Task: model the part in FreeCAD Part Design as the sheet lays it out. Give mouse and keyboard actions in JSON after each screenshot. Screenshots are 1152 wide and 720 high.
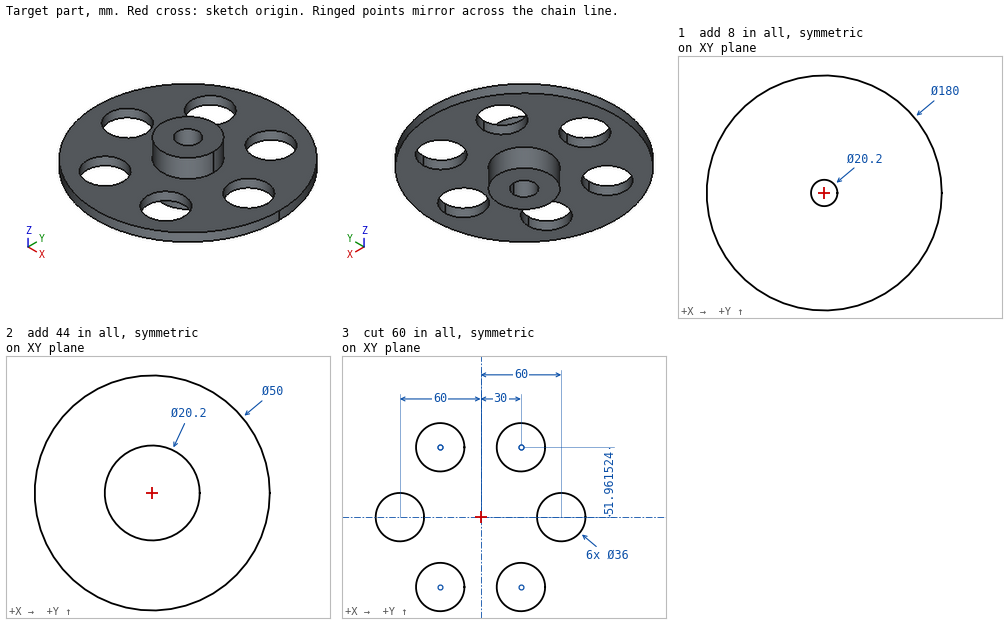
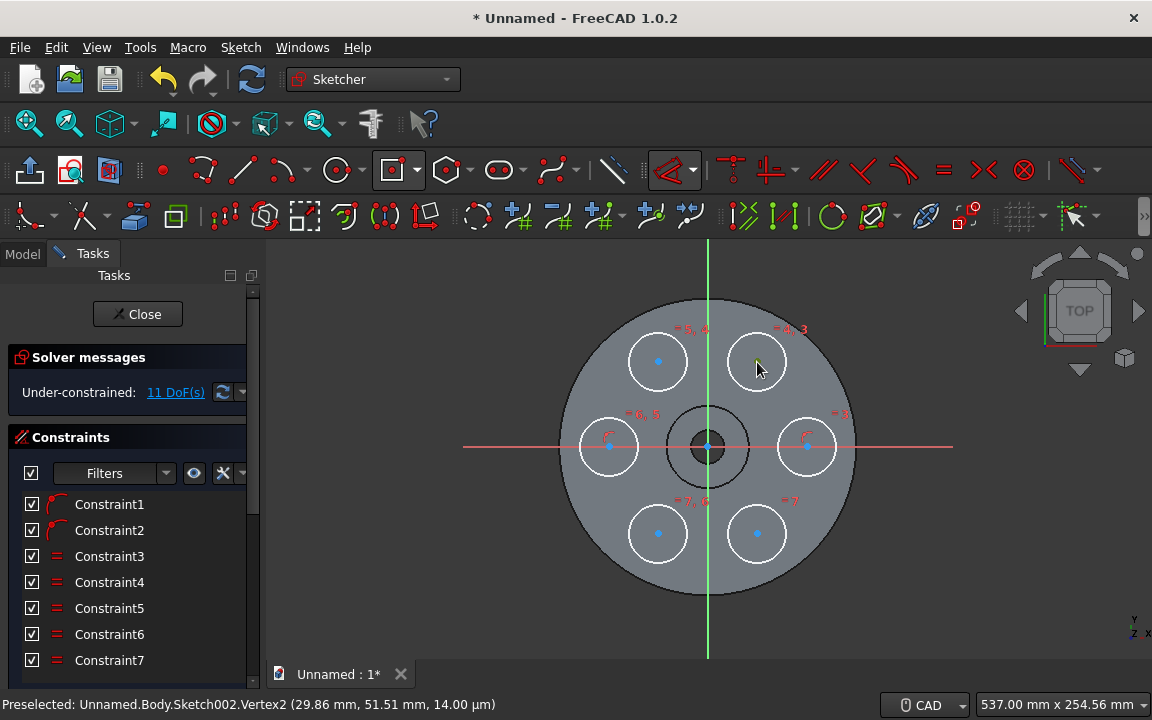
{"action": "left_click", "coordinate": [658, 362]}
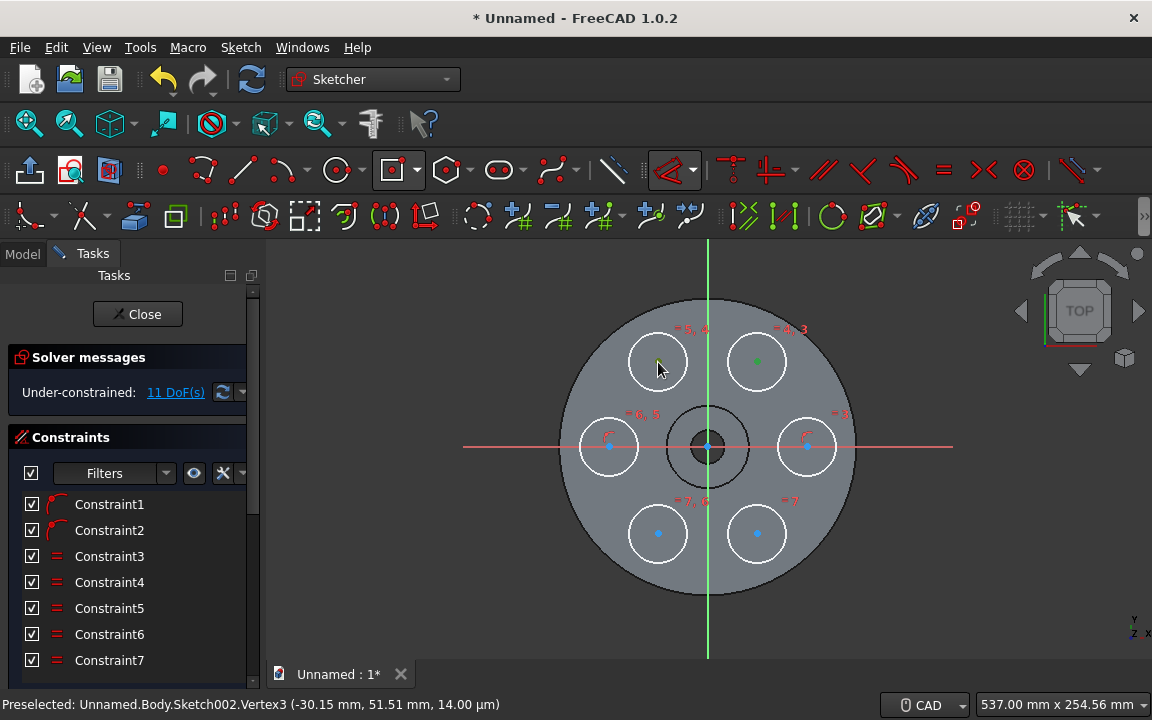
{"action": "left_click", "coordinate": [708, 605]}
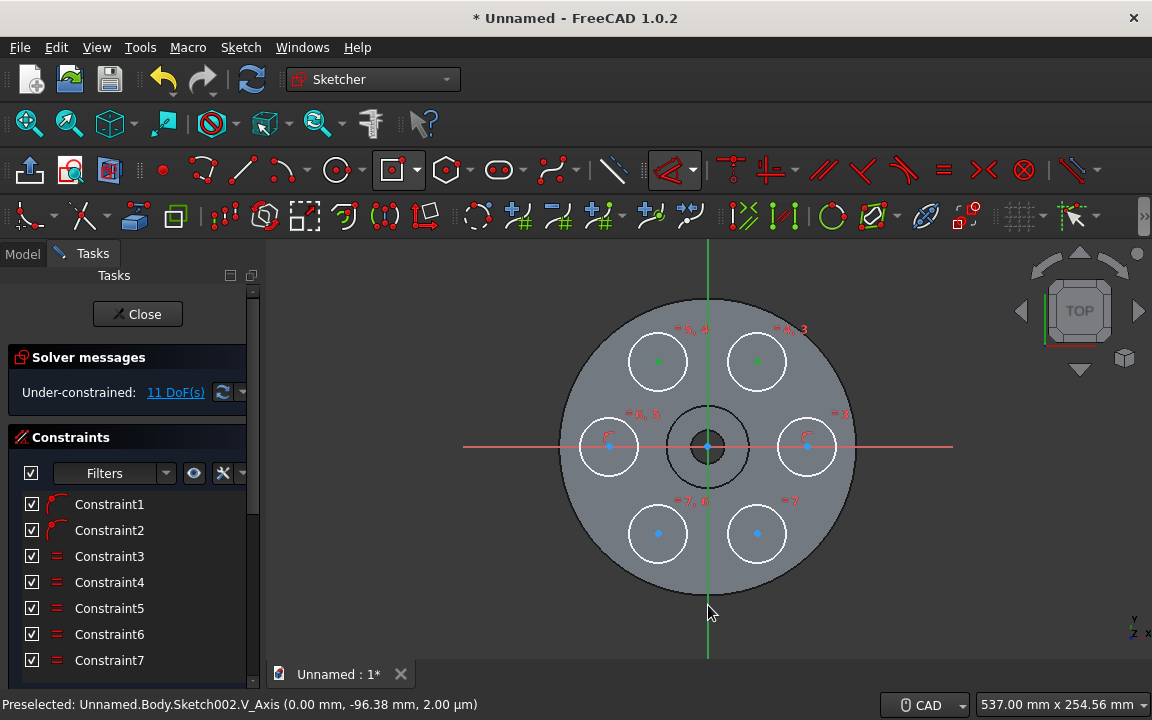
{"action": "key", "text": "s"}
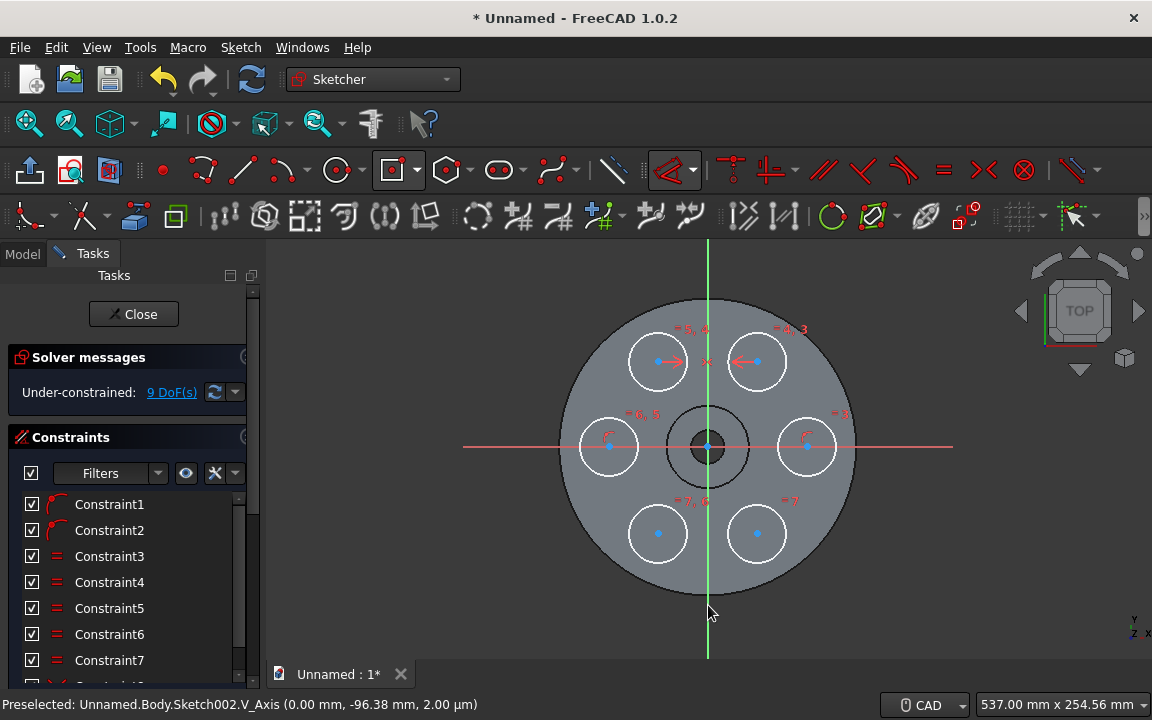
{"action": "left_click", "coordinate": [658, 362]}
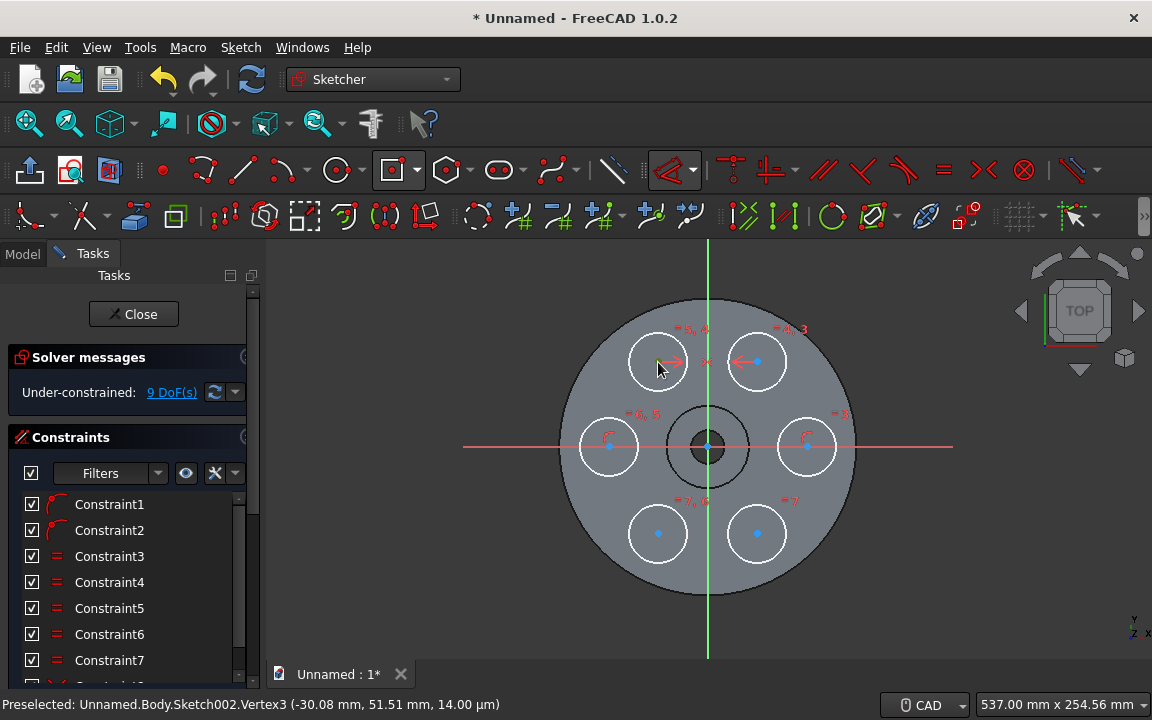
{"action": "left_click", "coordinate": [658, 534]}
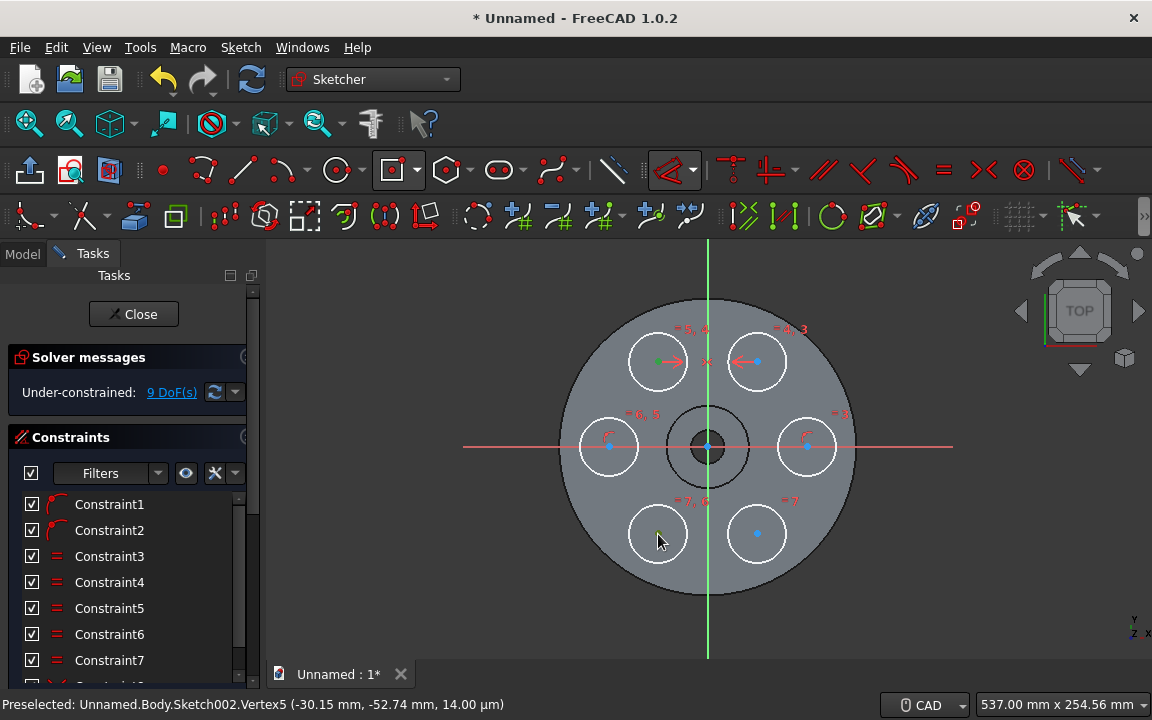
{"action": "left_click", "coordinate": [492, 447]}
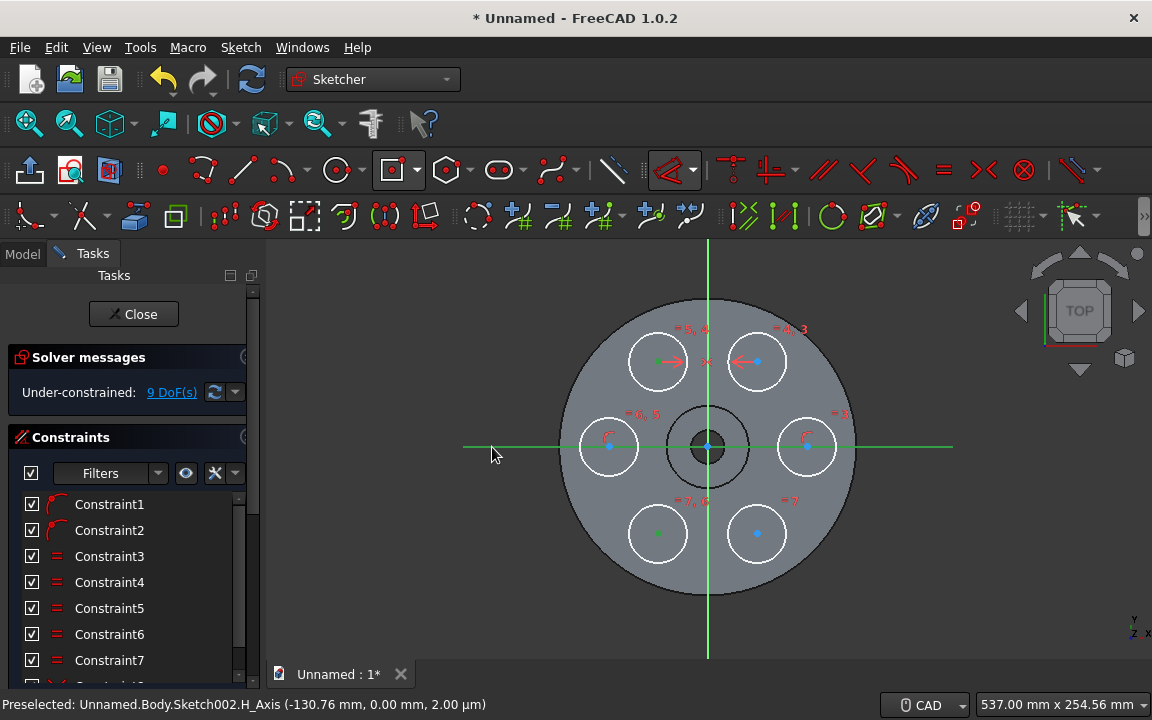
{"action": "key", "text": "s"}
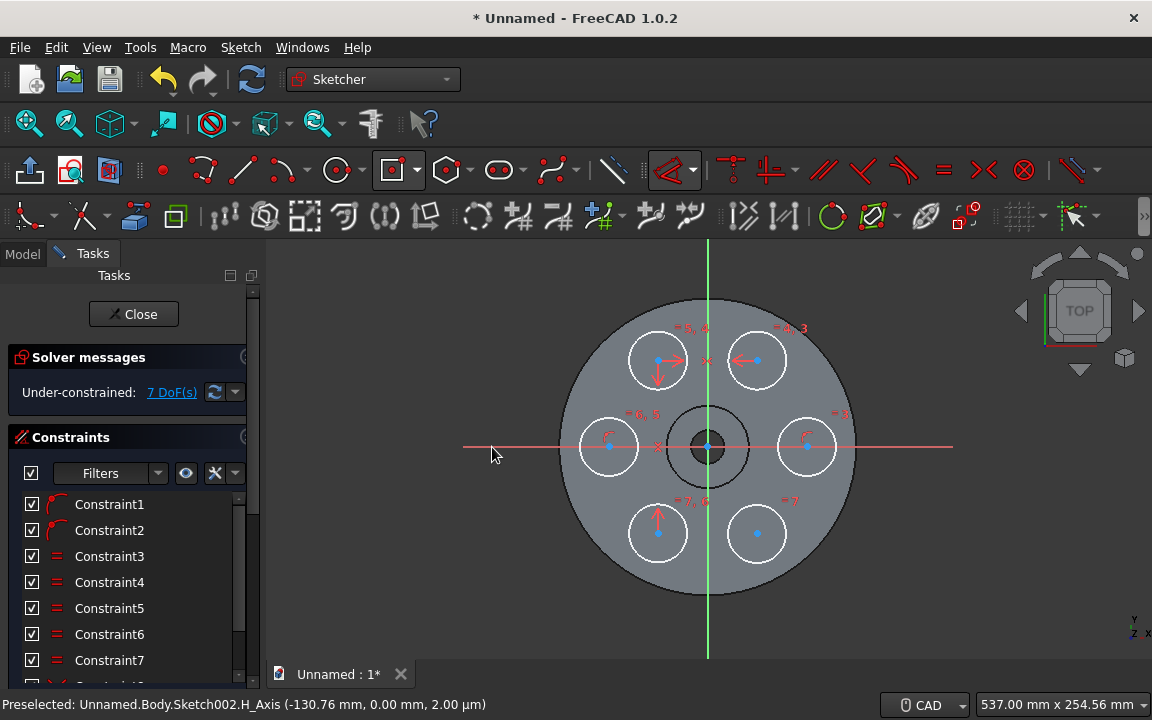
{"action": "left_click", "coordinate": [757, 361]}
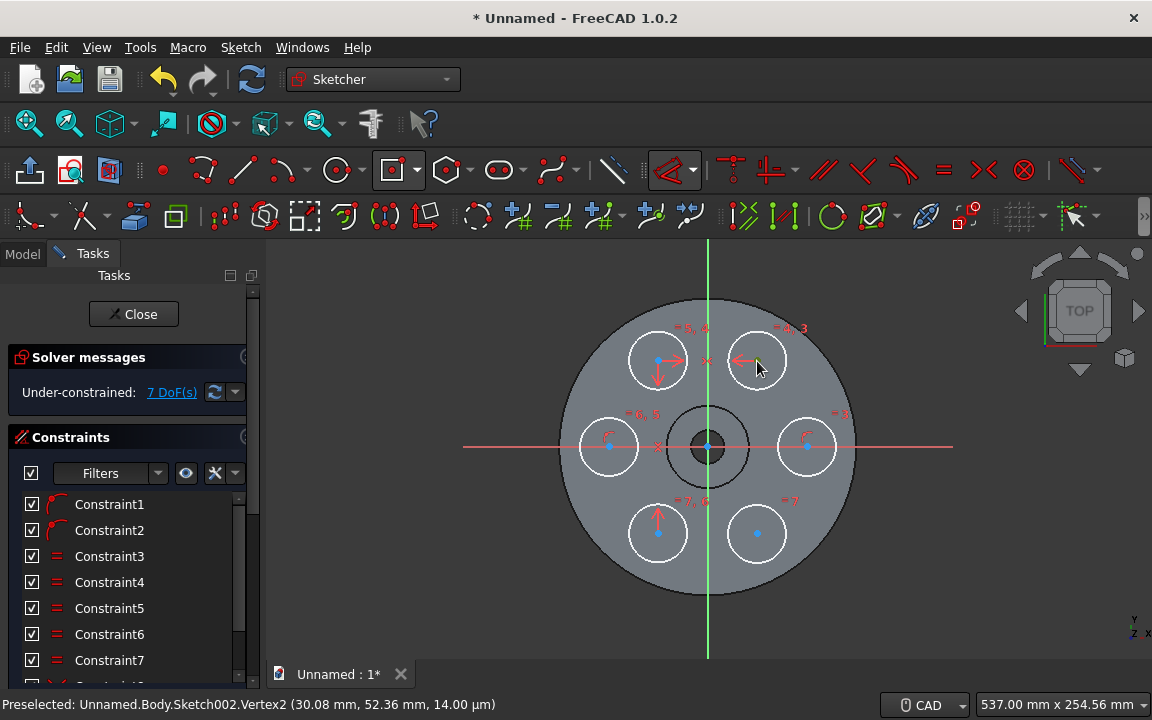
{"action": "left_click", "coordinate": [757, 534]}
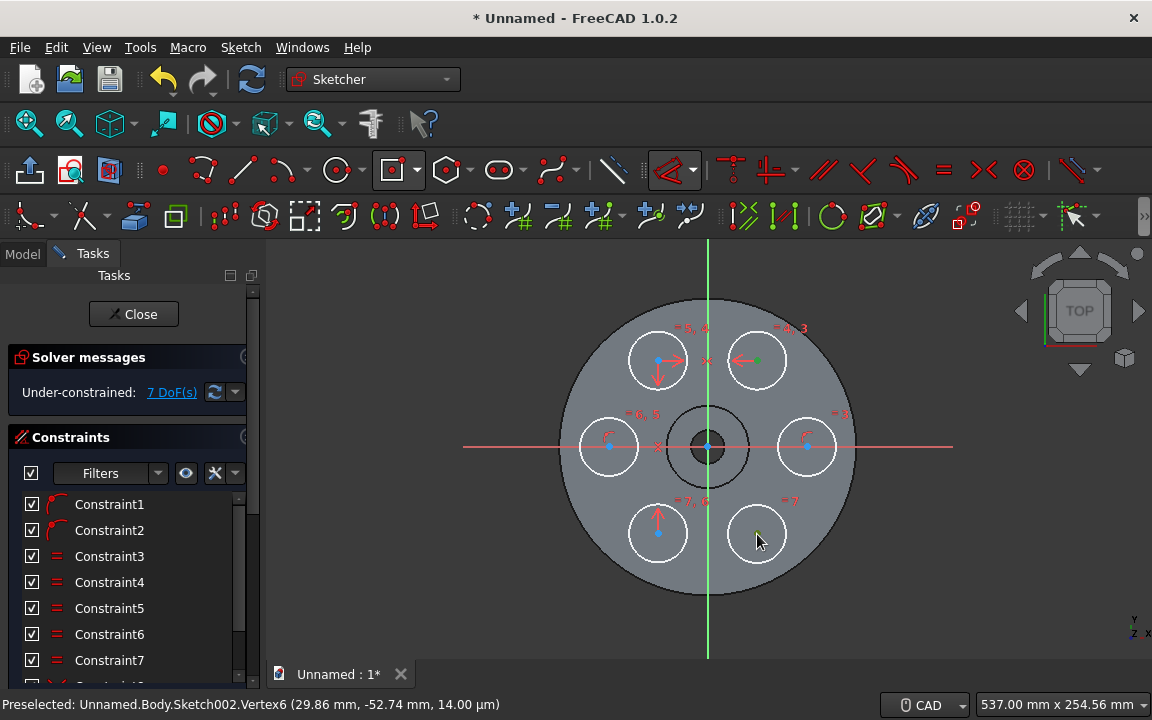
{"action": "left_click", "coordinate": [492, 447]}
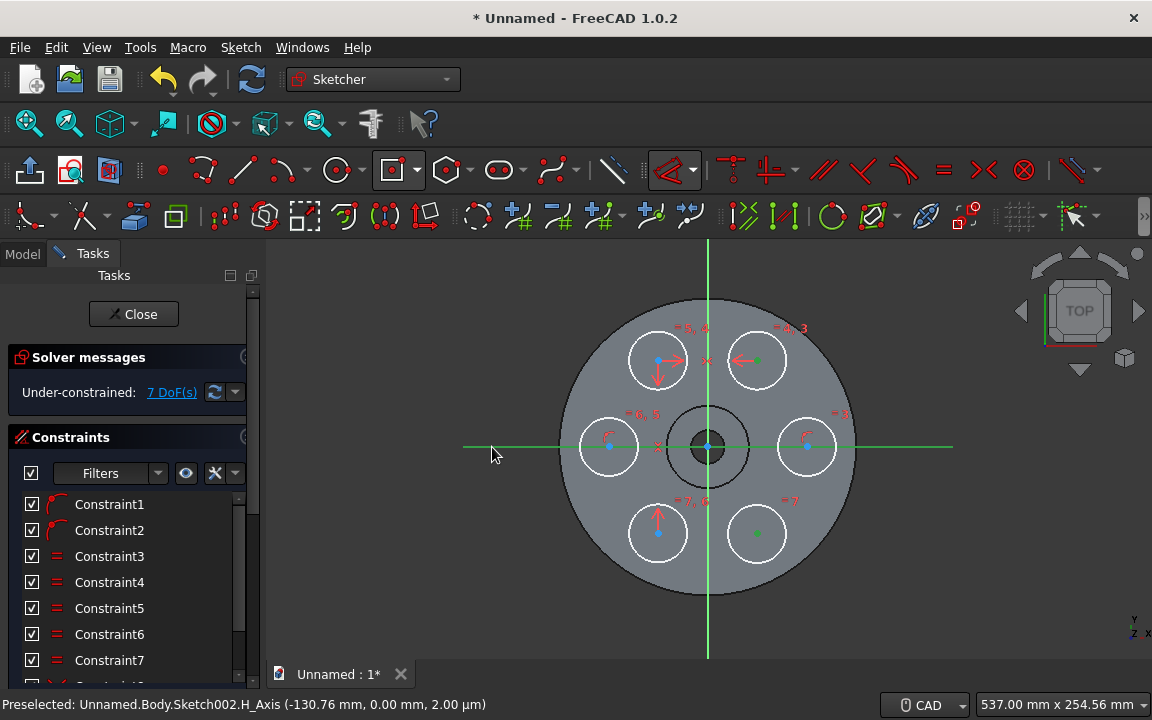
{"action": "left_click", "coordinate": [984, 170]}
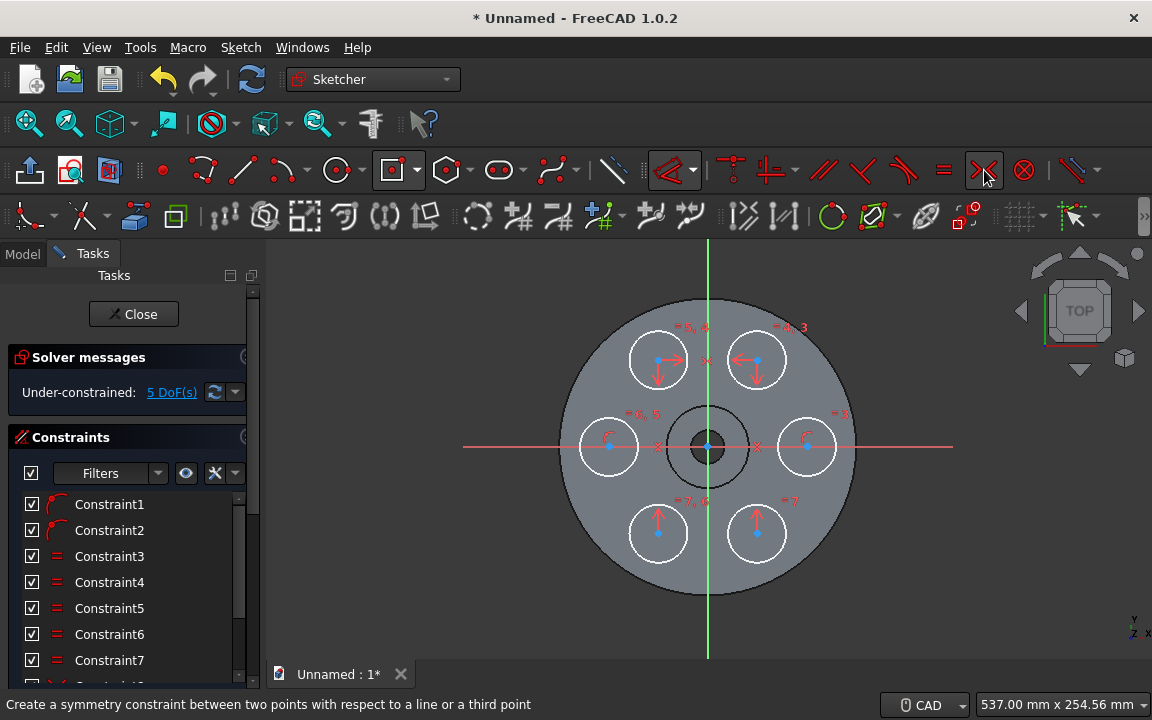
{"action": "left_click", "coordinate": [827, 426]}